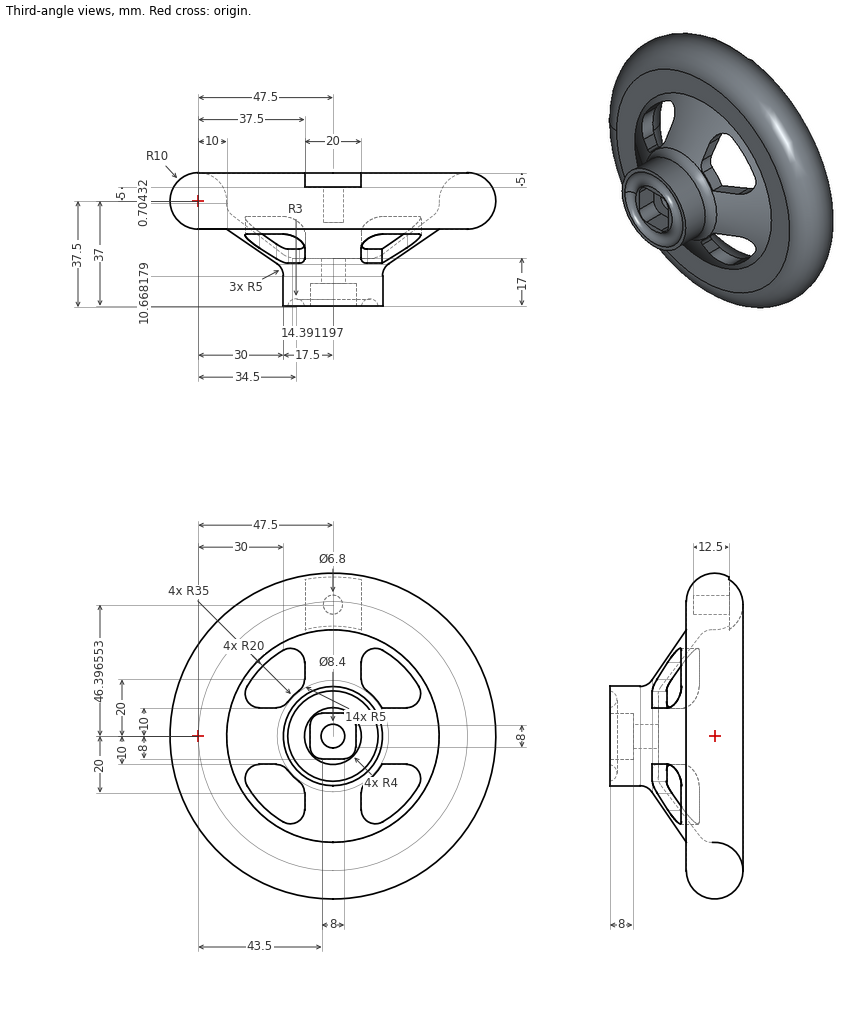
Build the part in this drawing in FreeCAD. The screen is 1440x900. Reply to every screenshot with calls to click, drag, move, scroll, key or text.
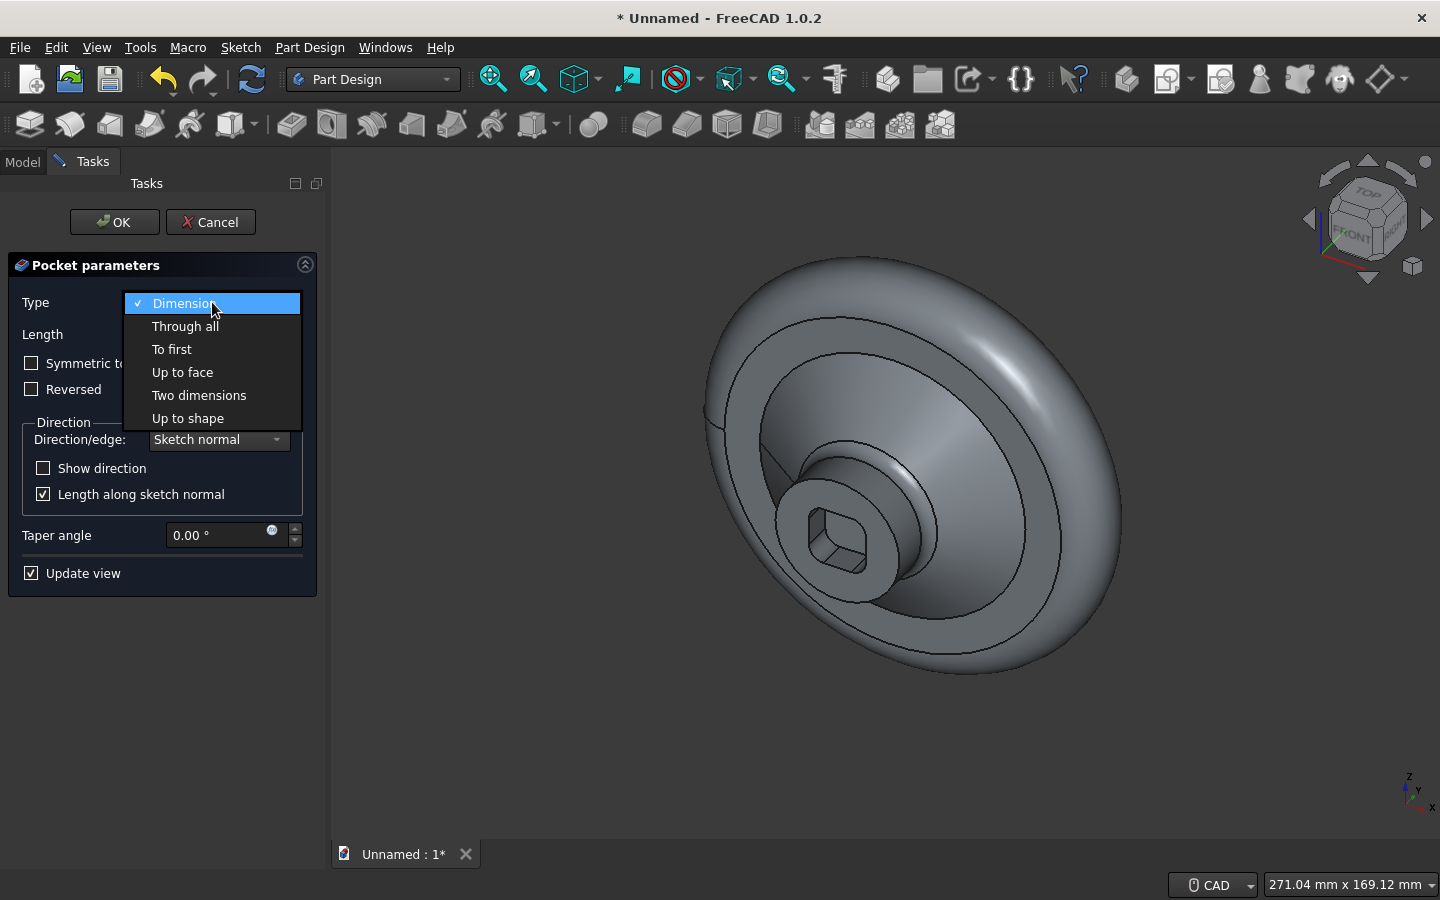
click(212, 326)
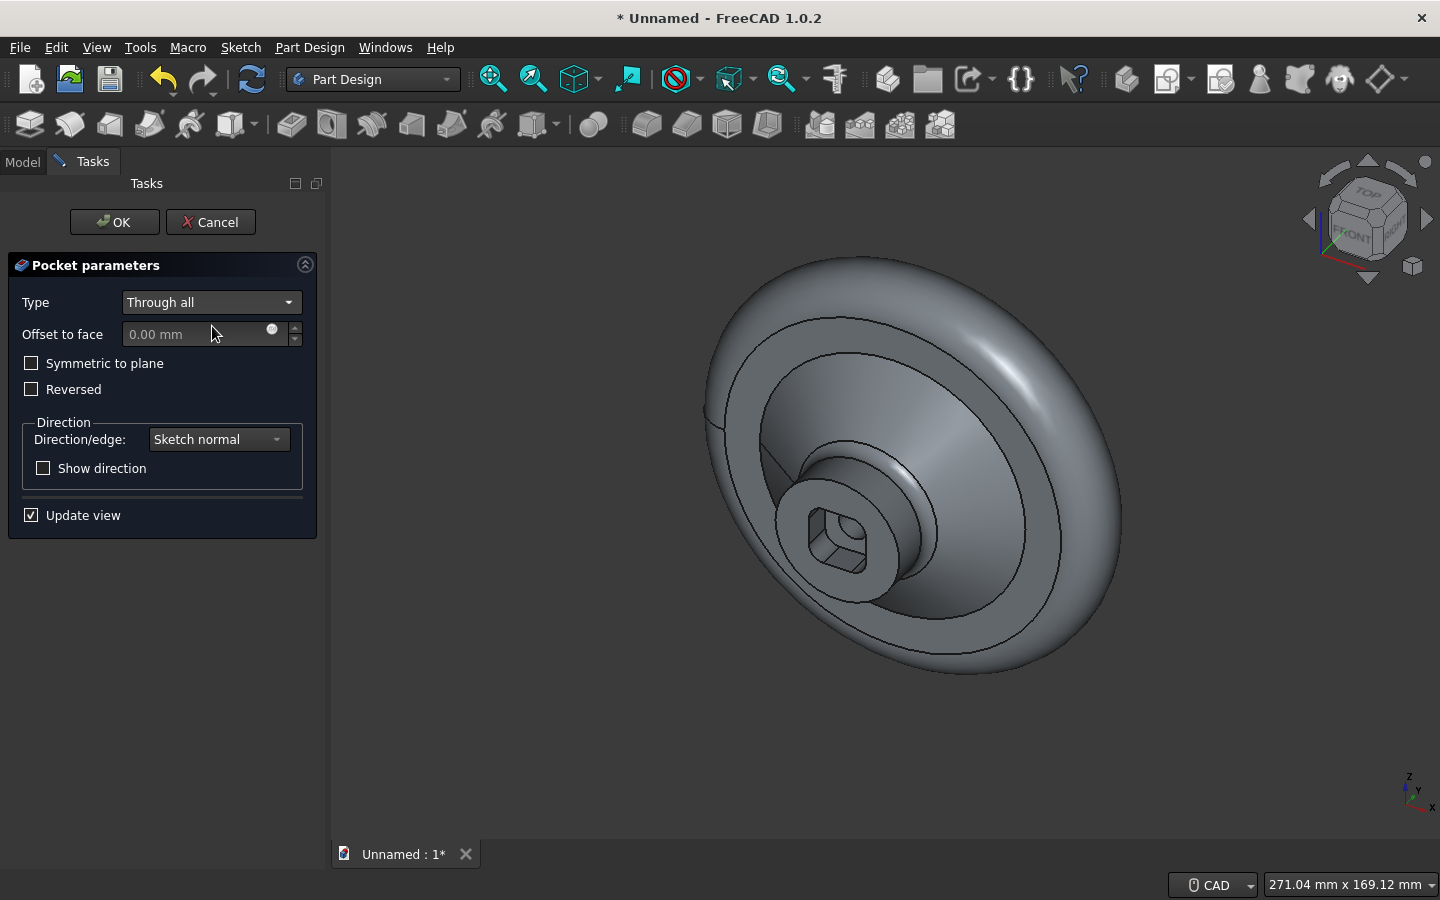
click(115, 222)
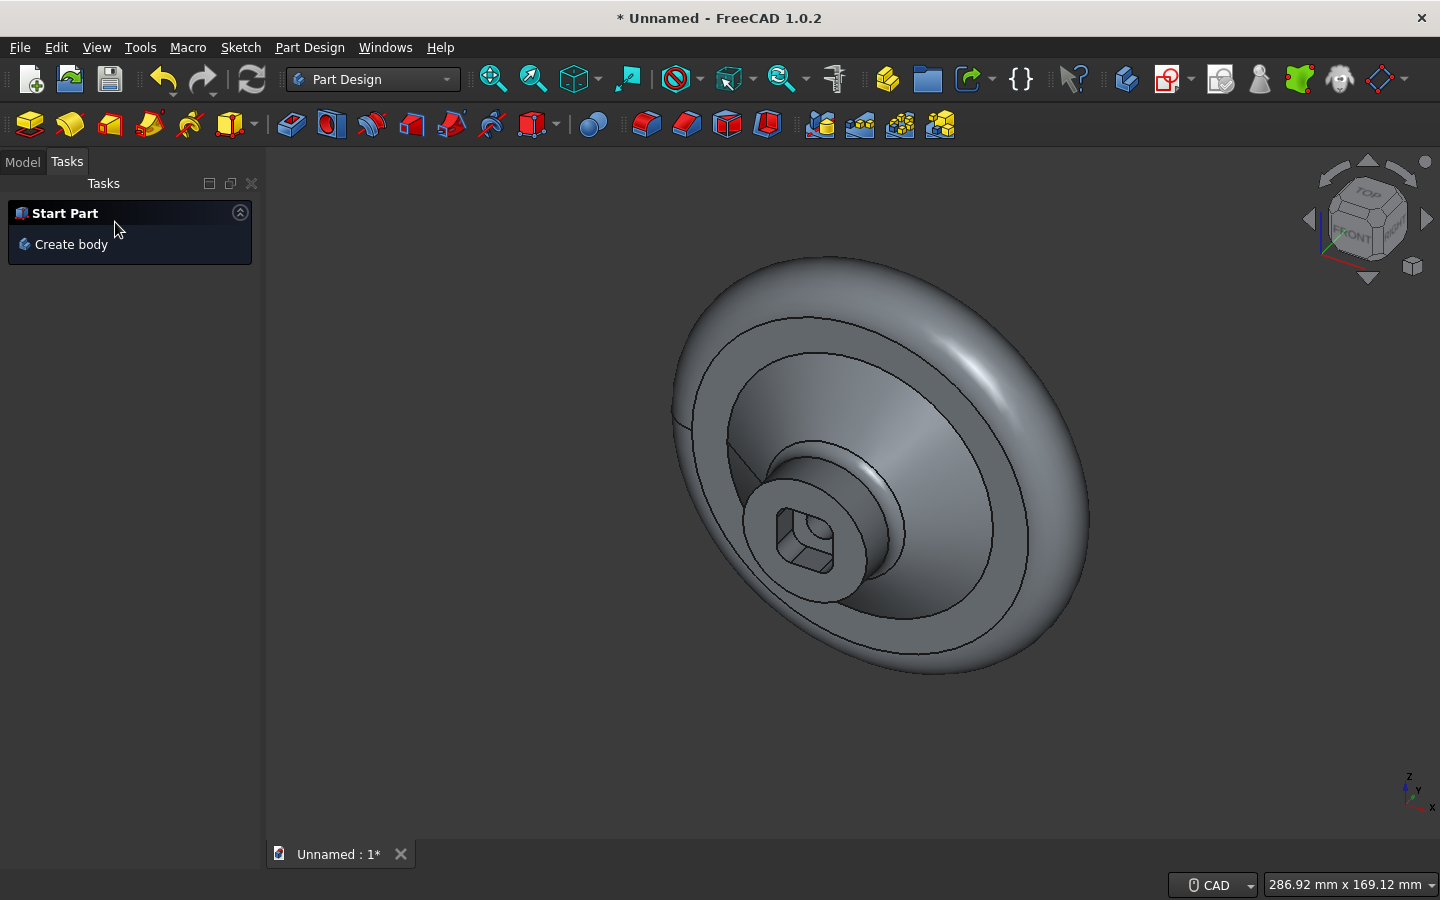
click(1168, 80)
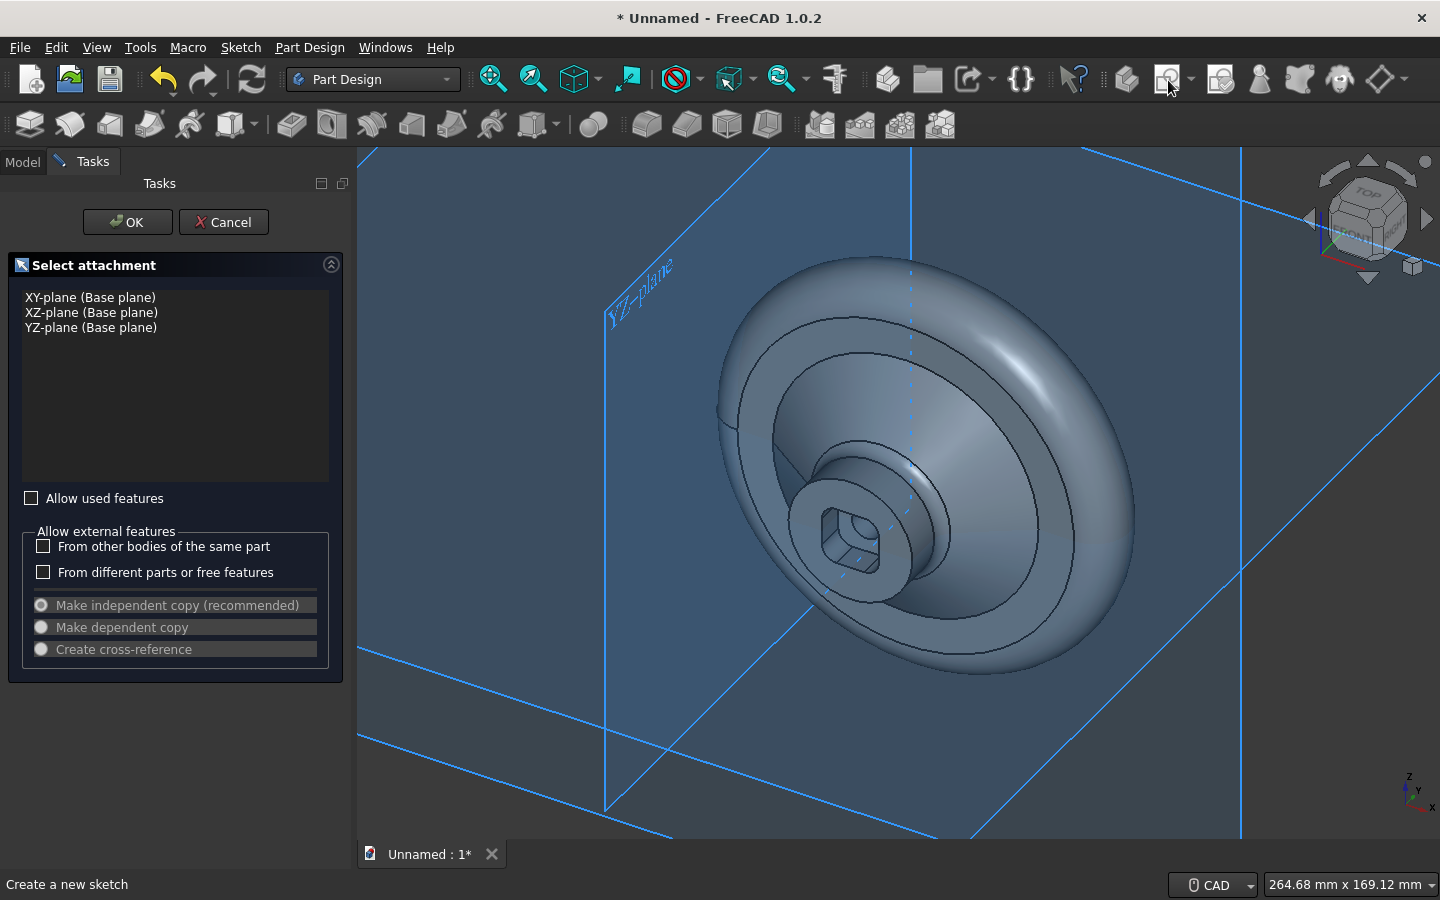
click(82, 298)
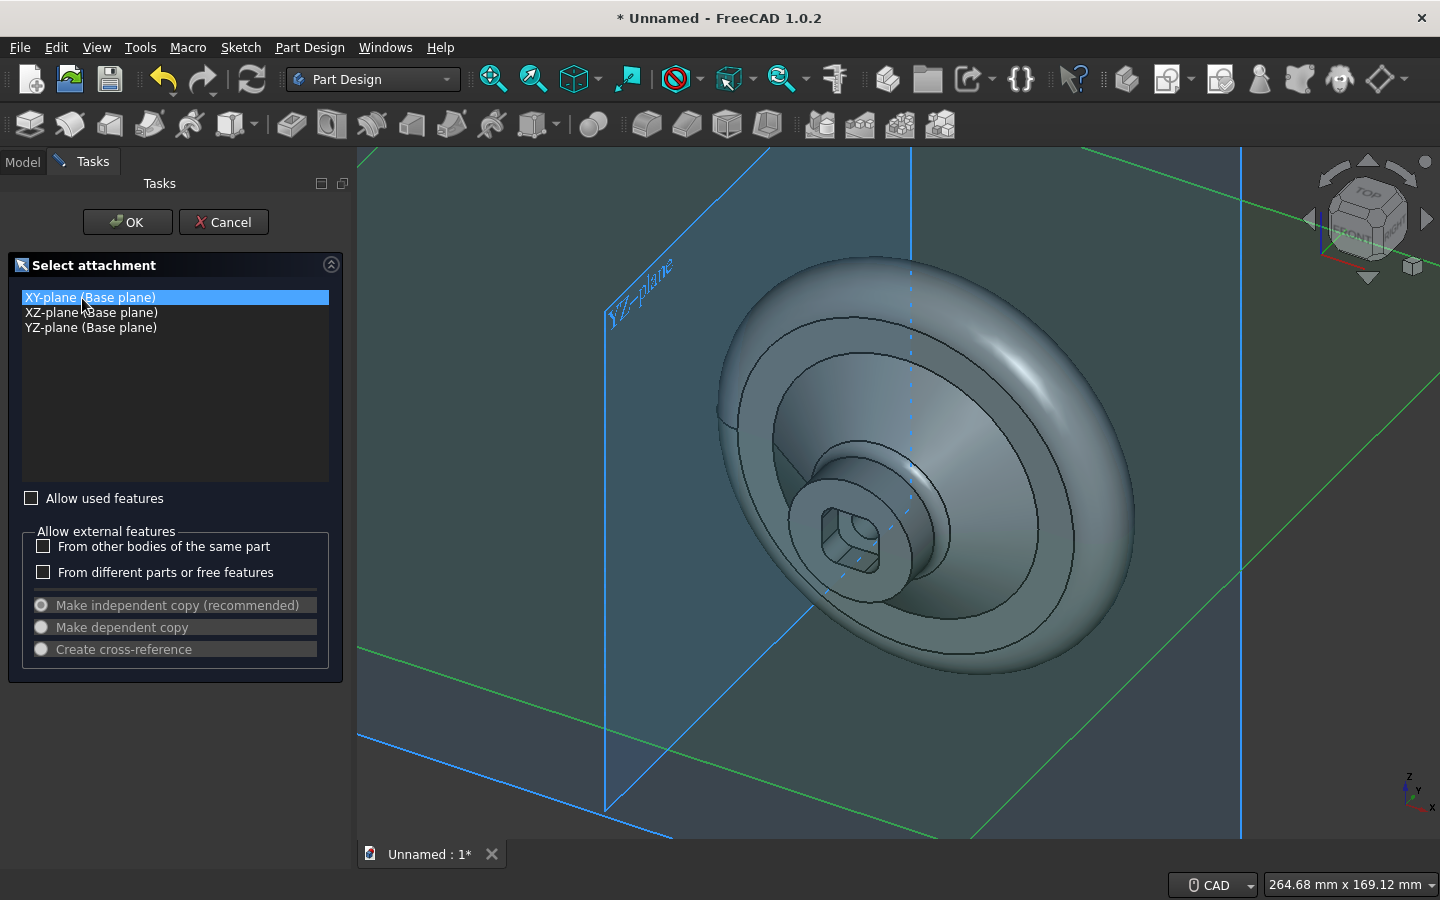
click(128, 222)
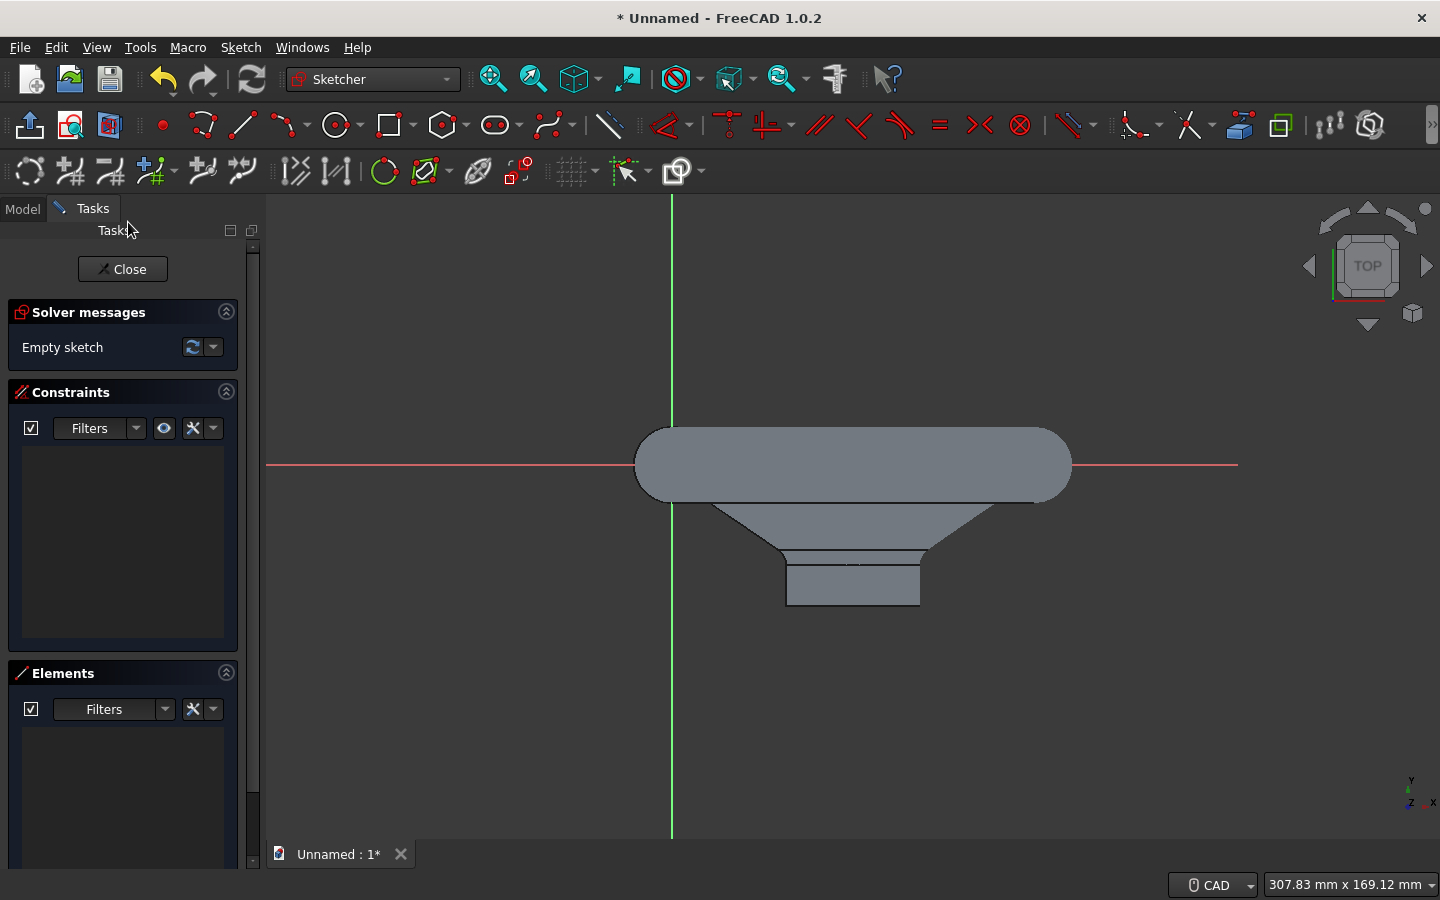
click(110, 126)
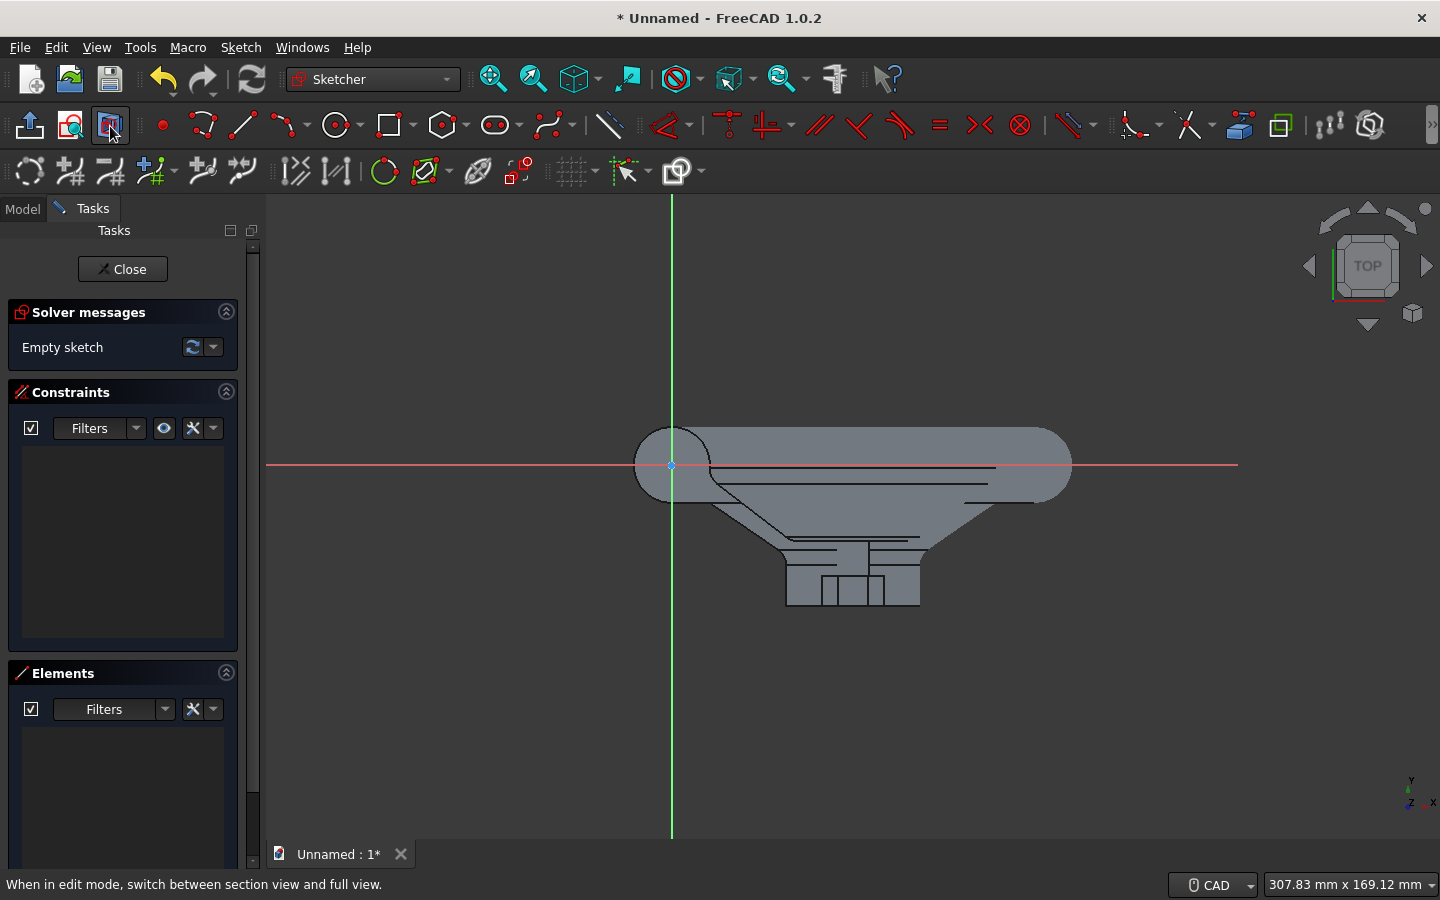
scroll(826, 610, up, 12)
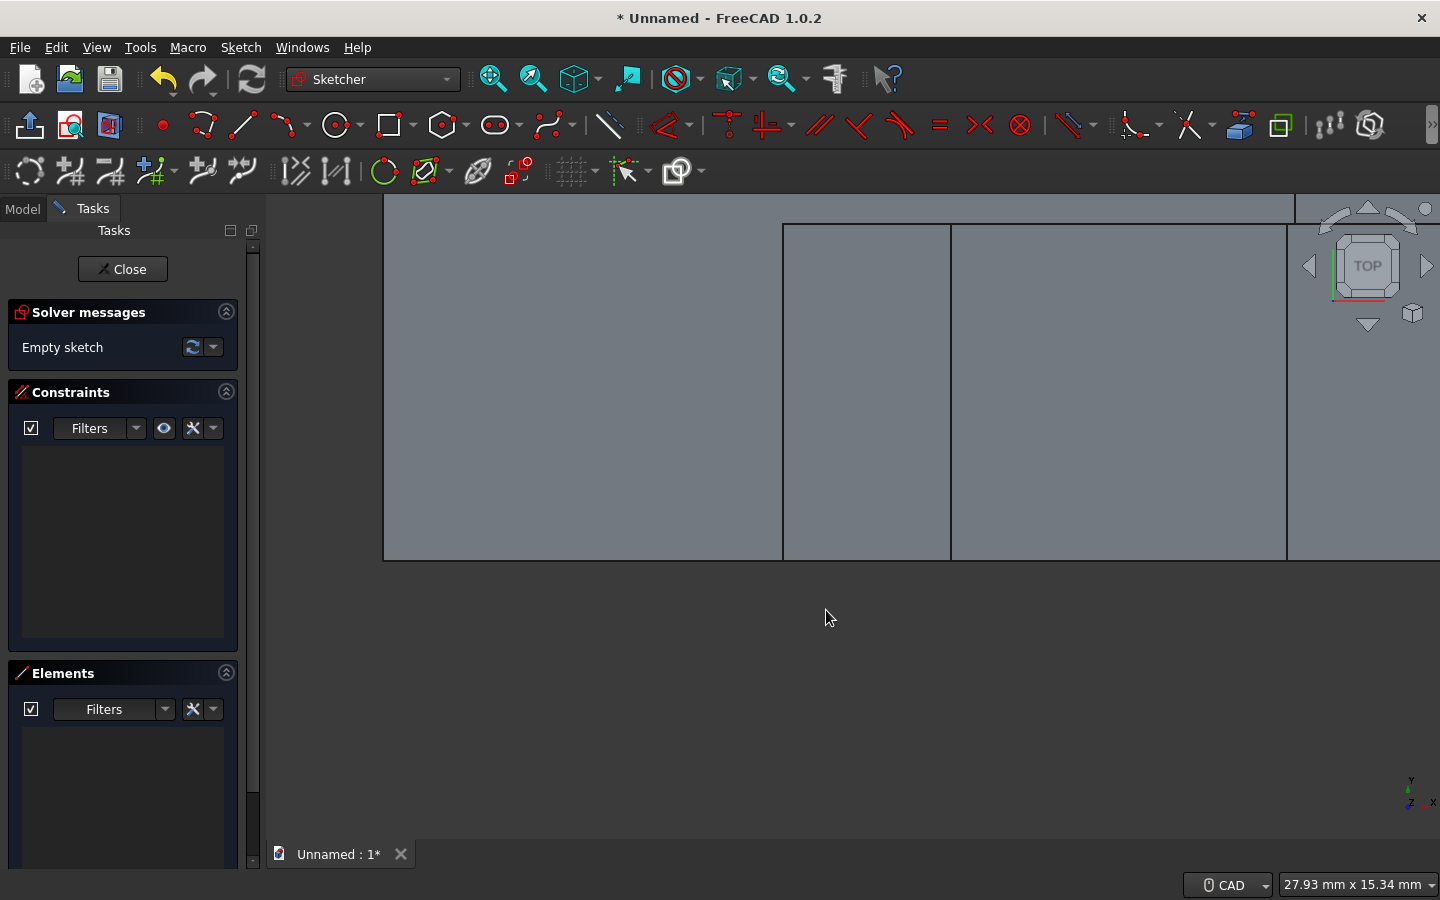
click(244, 126)